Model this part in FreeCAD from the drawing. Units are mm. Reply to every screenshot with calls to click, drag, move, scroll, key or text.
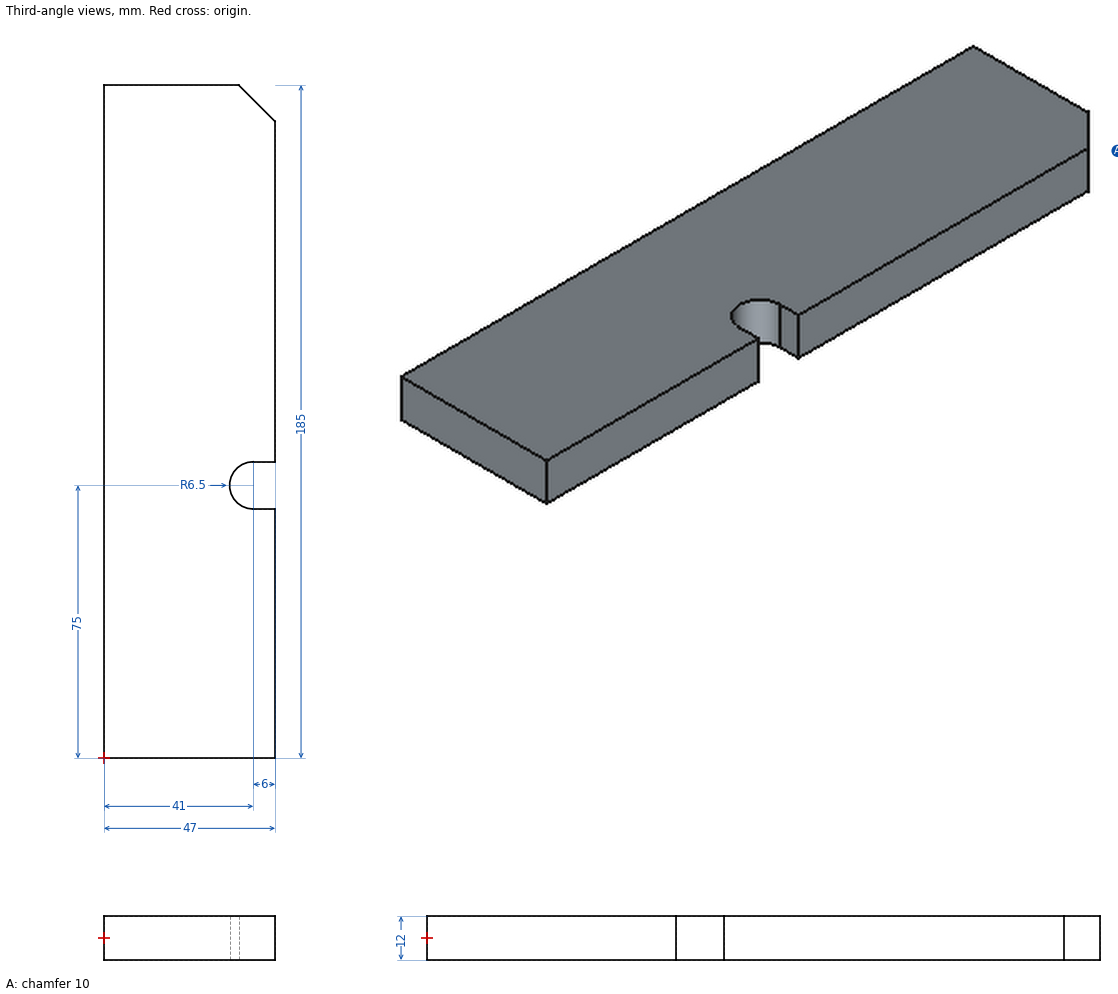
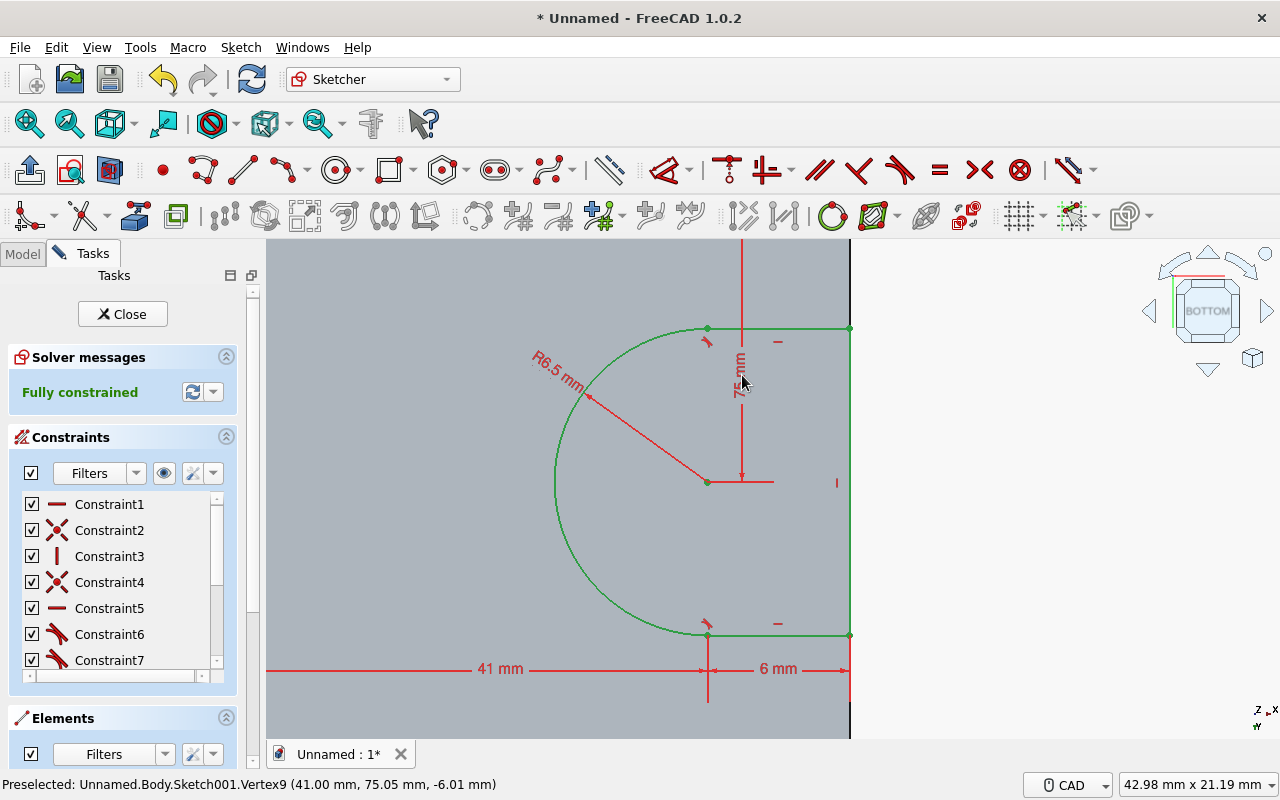
click(123, 314)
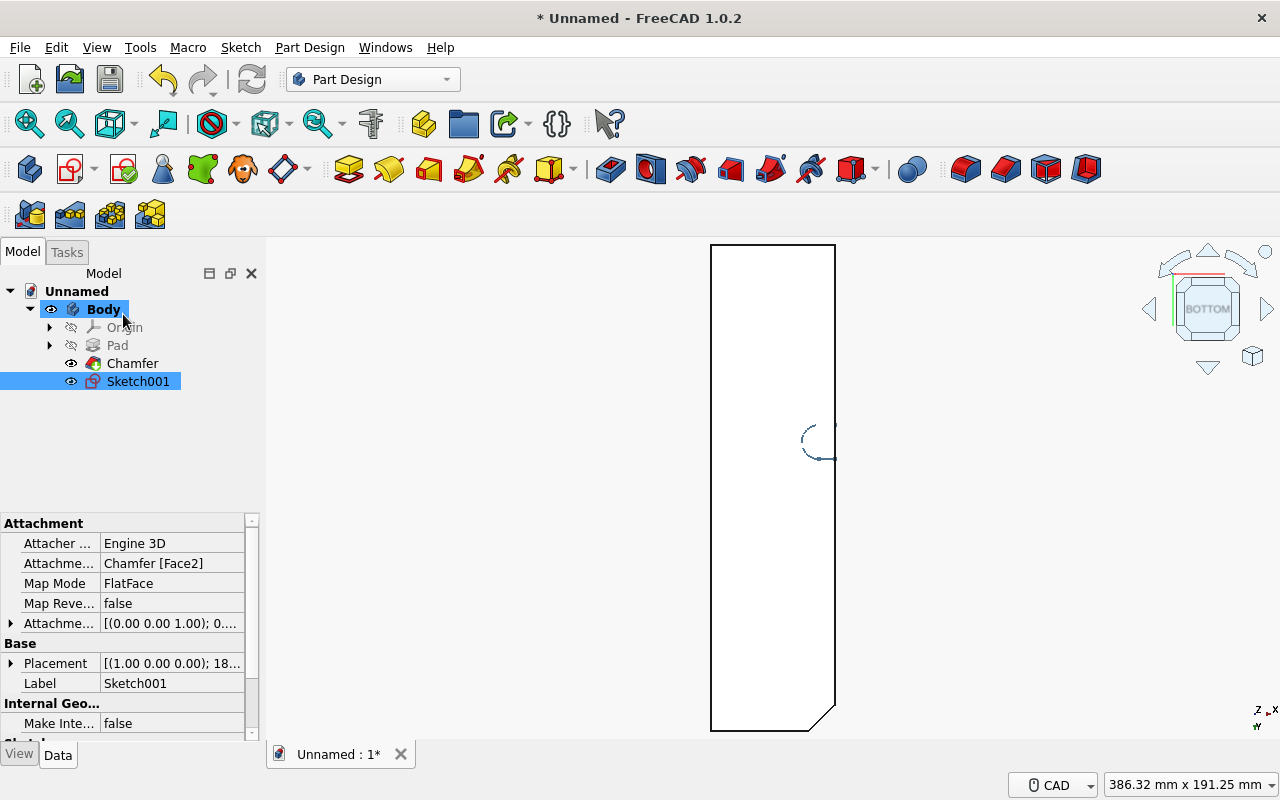
click(612, 170)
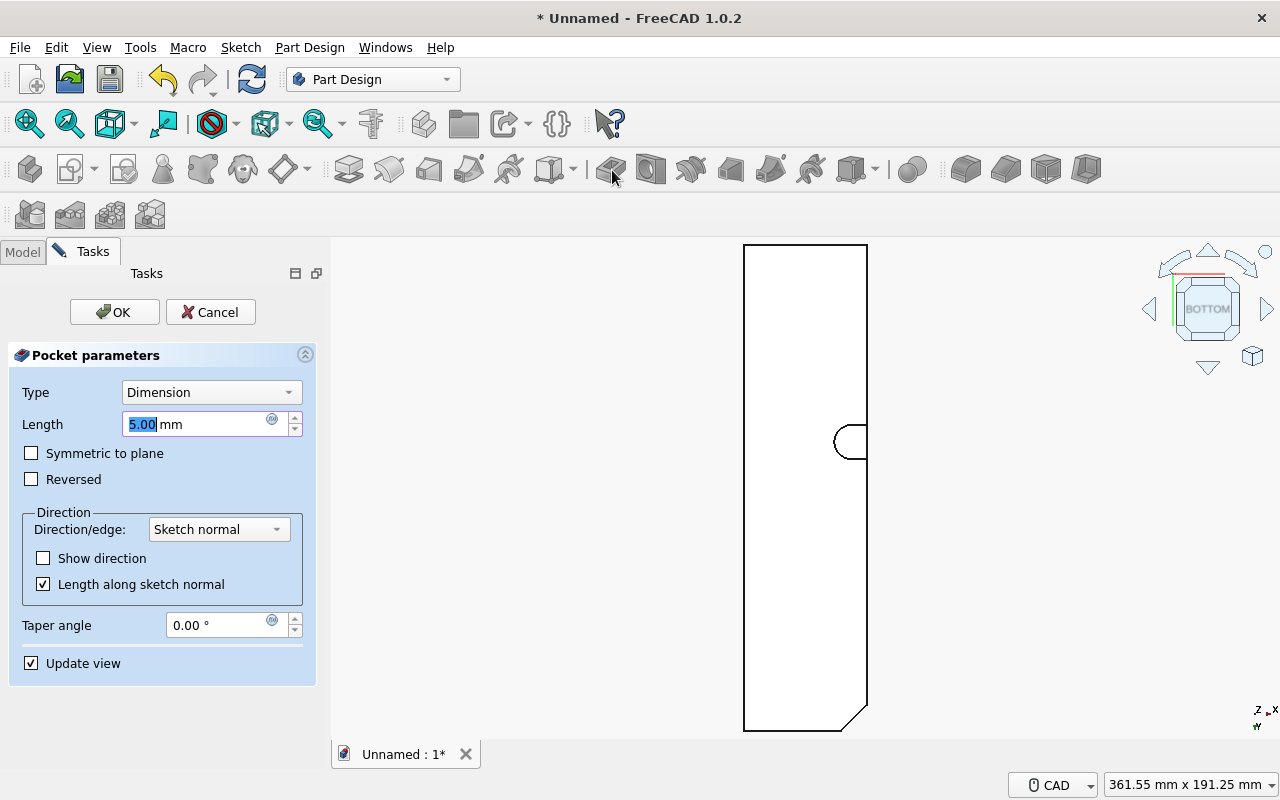
click(212, 392)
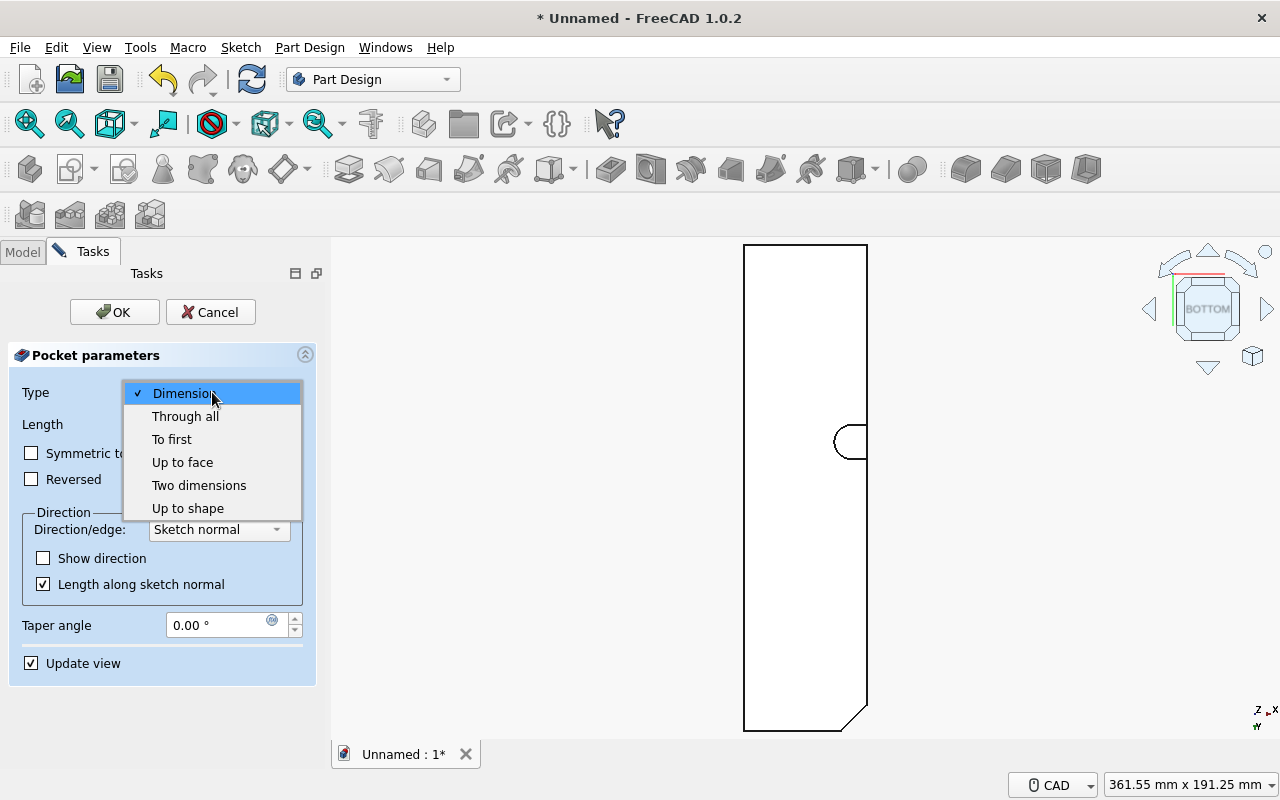
click(212, 440)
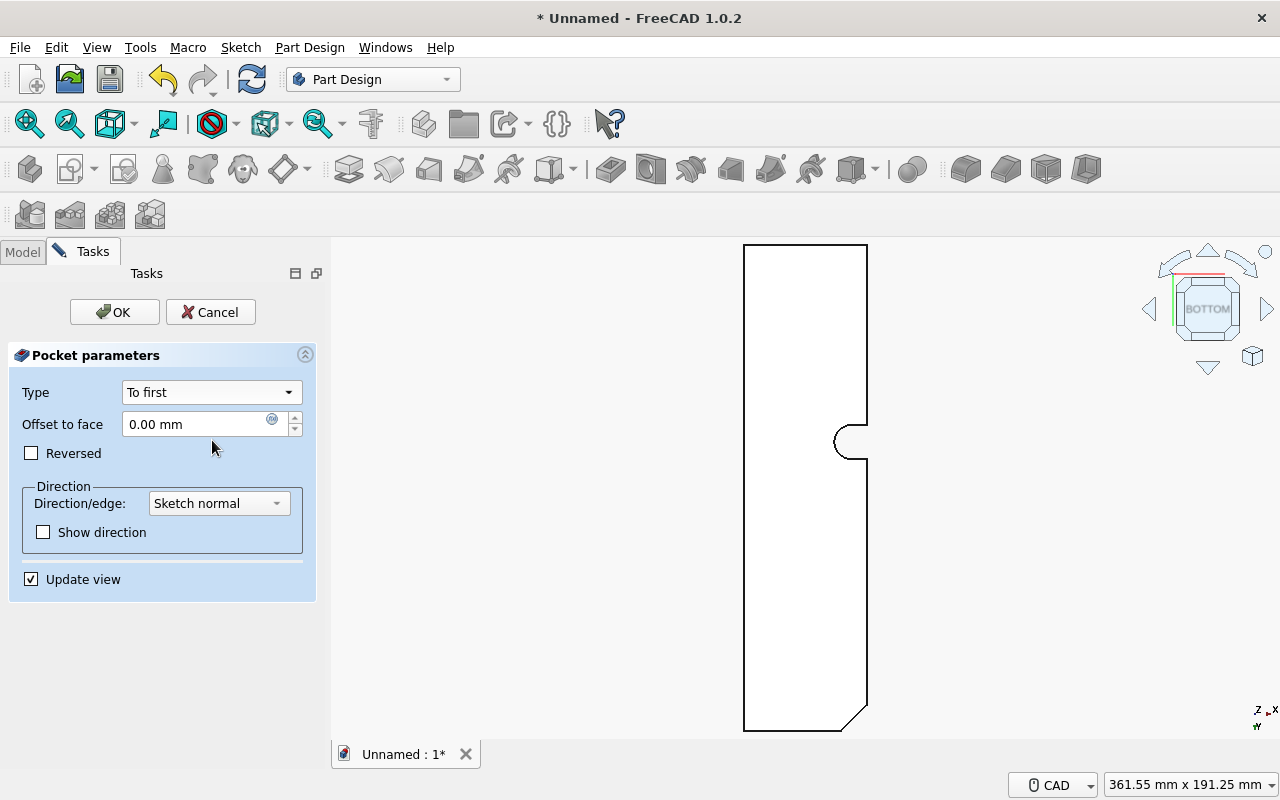
click(115, 312)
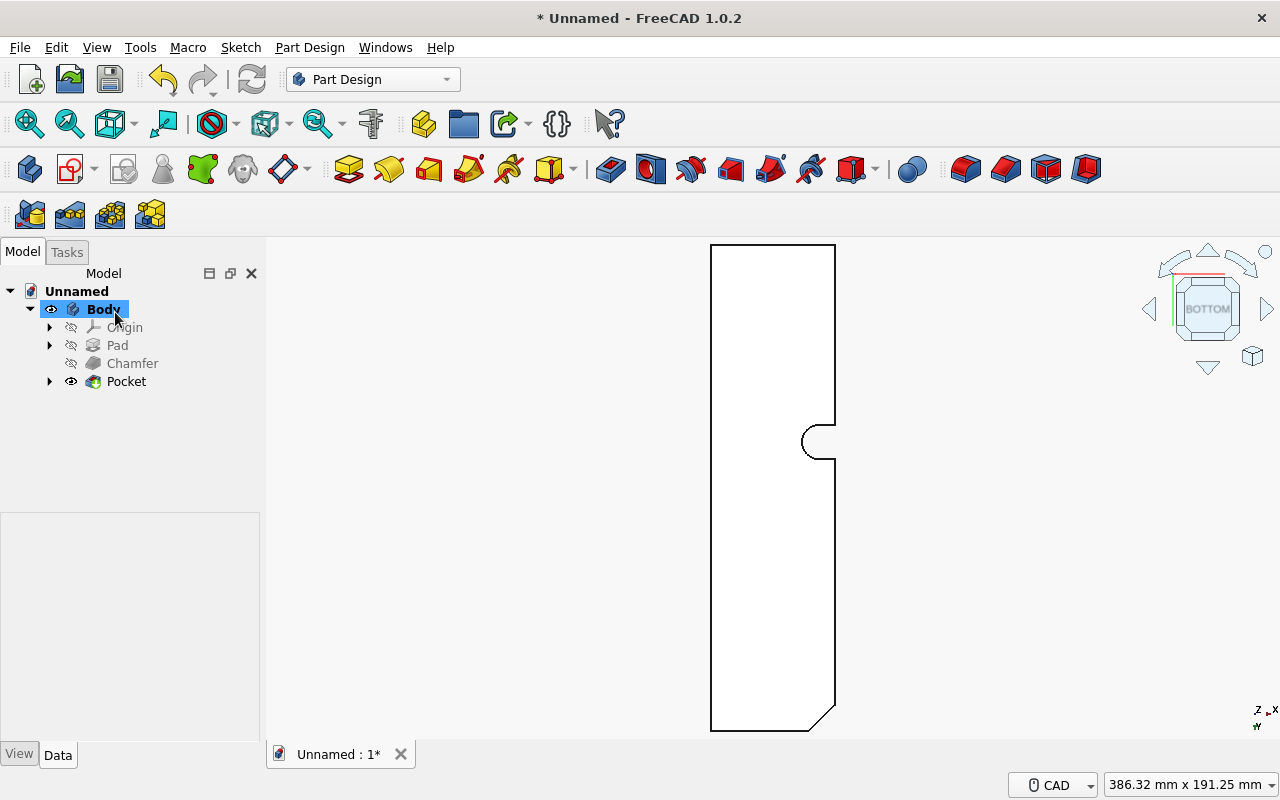
key(0)